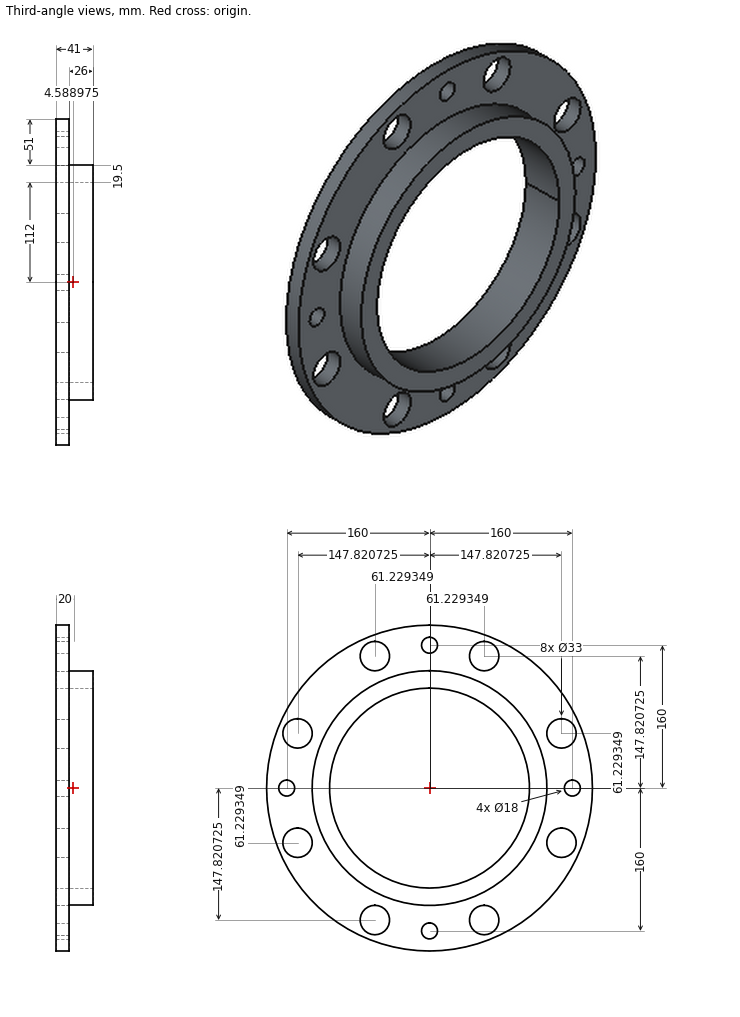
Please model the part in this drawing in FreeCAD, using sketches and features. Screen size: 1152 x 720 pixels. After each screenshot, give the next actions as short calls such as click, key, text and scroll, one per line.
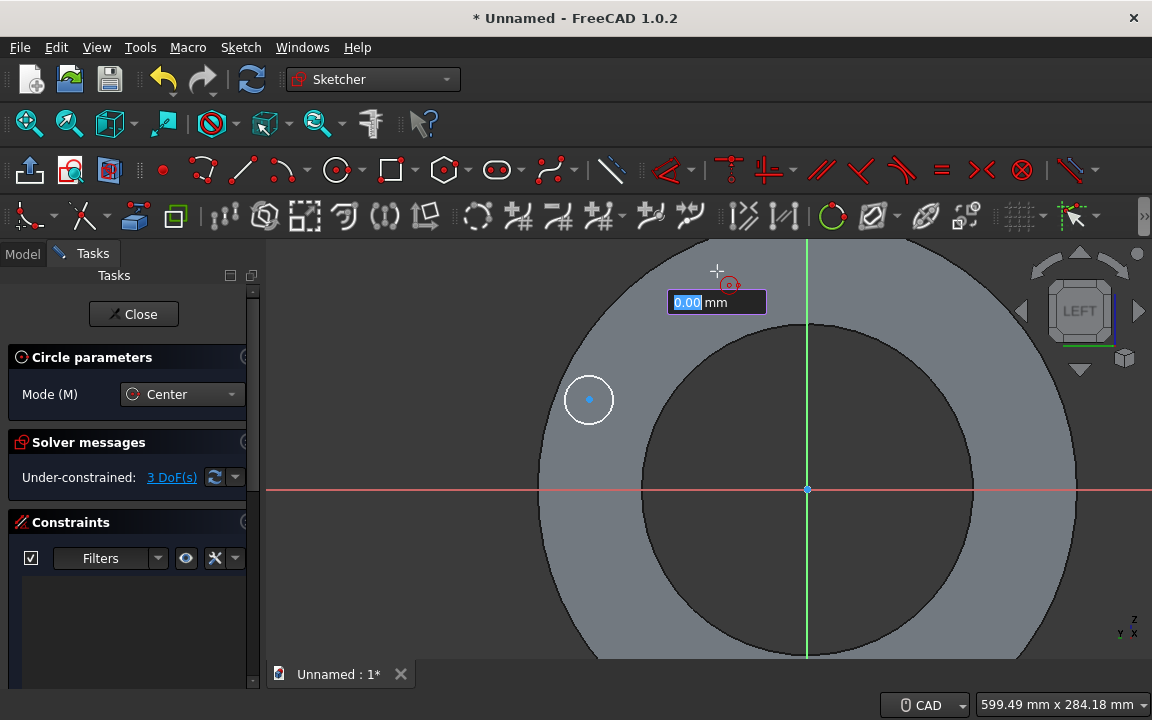
scroll(438, 399, down, 3)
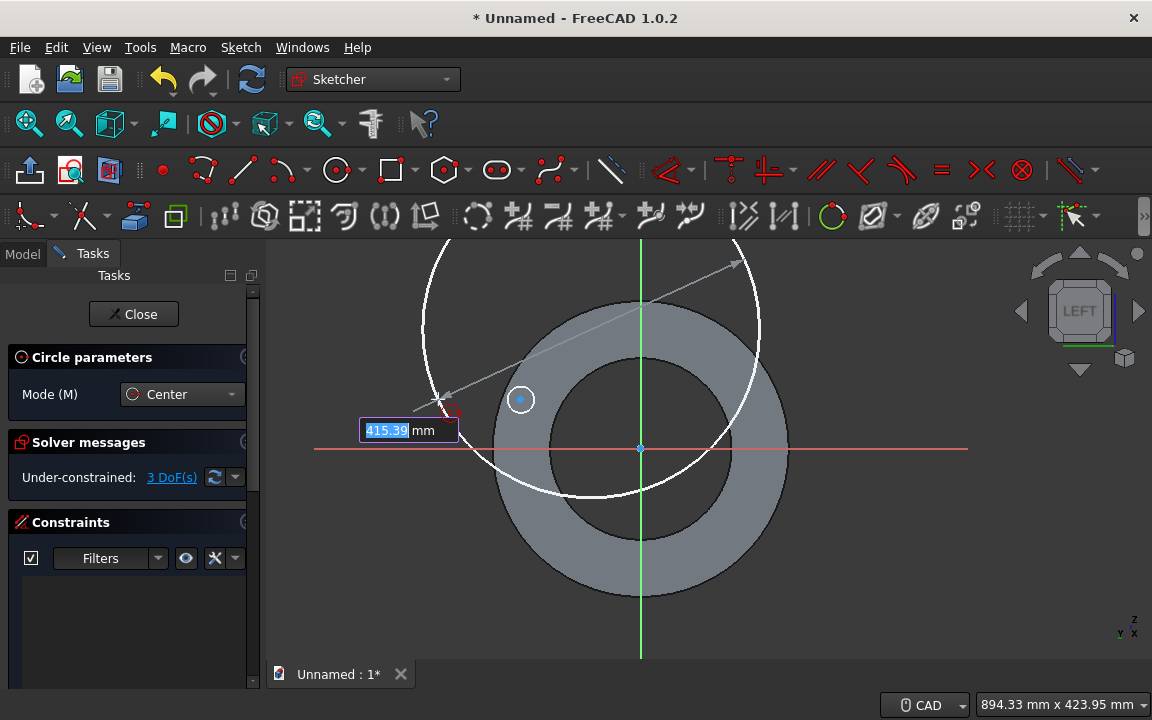
click(601, 320)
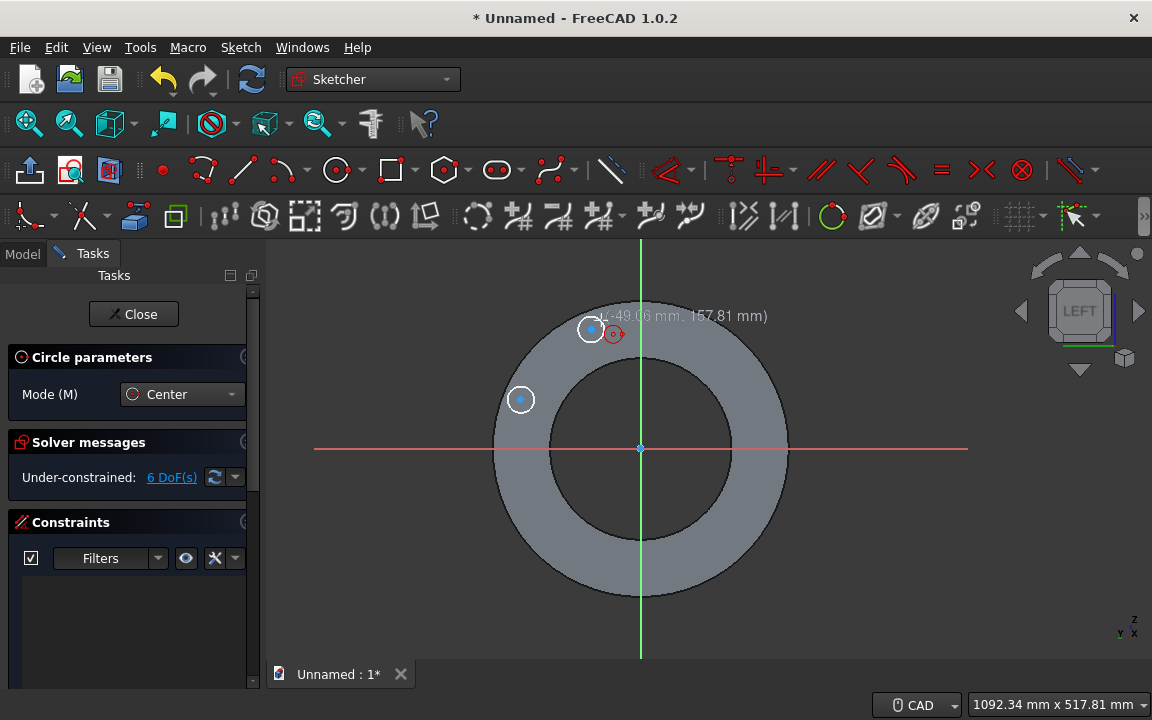
scroll(690, 329, up, 3)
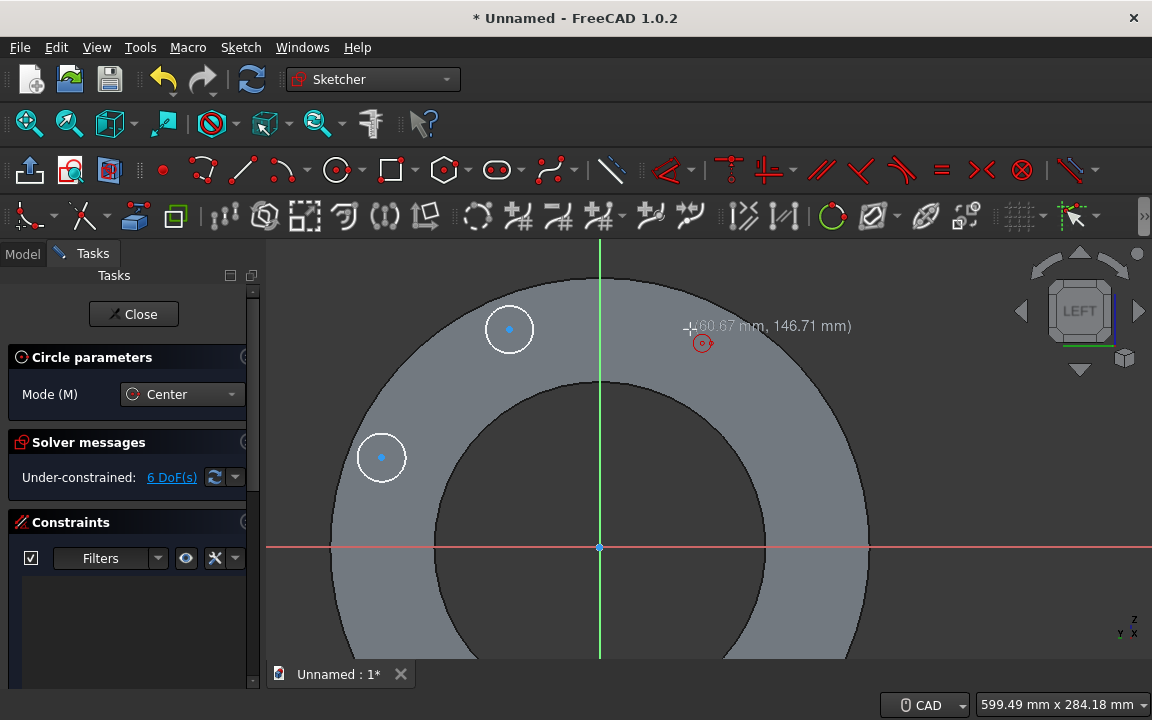
click(690, 329)
click(708, 312)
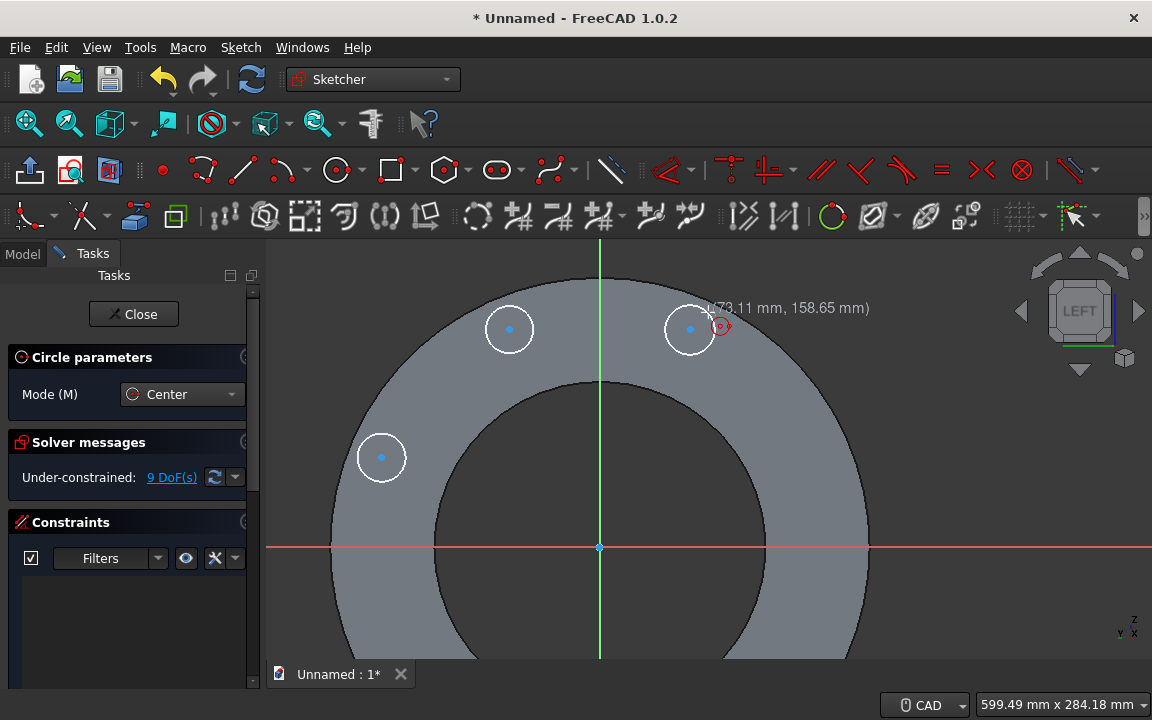
click(818, 457)
click(836, 440)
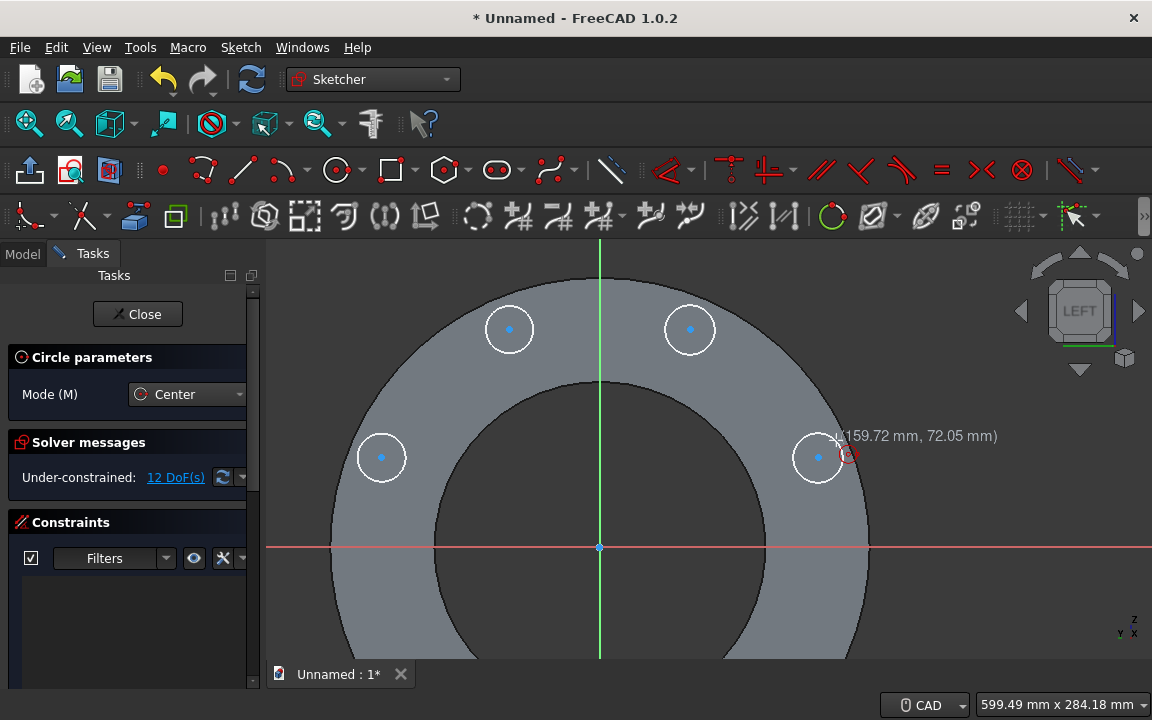
scroll(690, 329, down, 3)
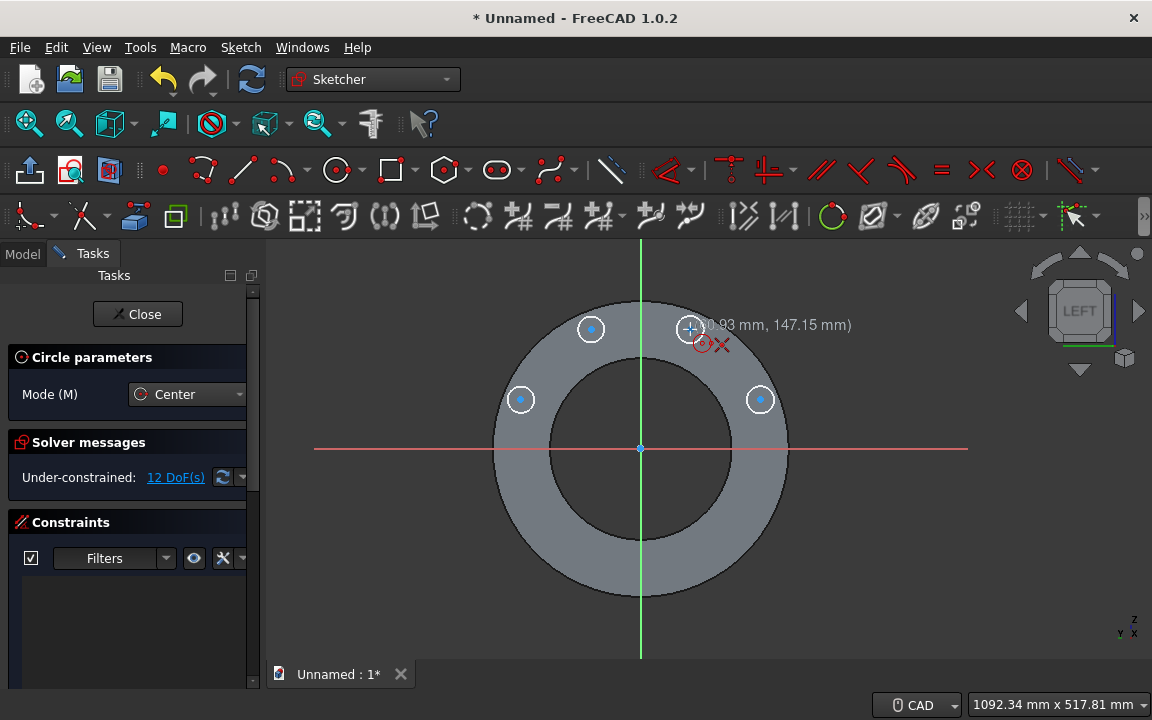
scroll(761, 499, up, 3)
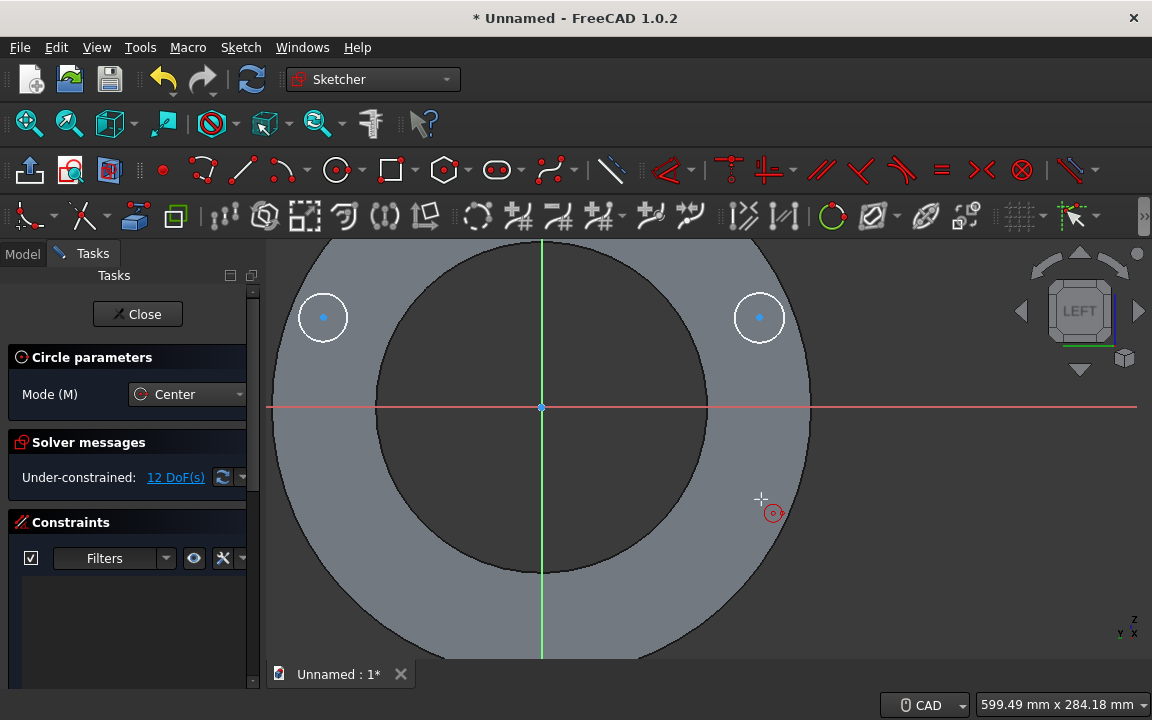
click(760, 498)
click(777, 481)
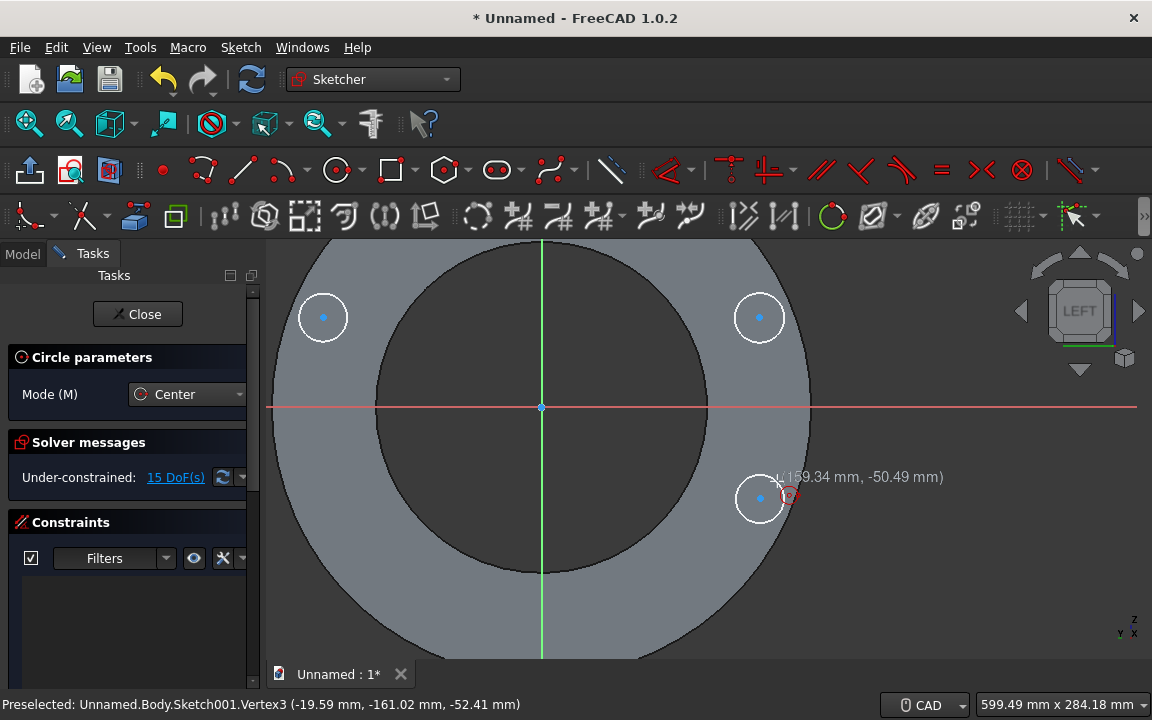
click(632, 626)
click(649, 609)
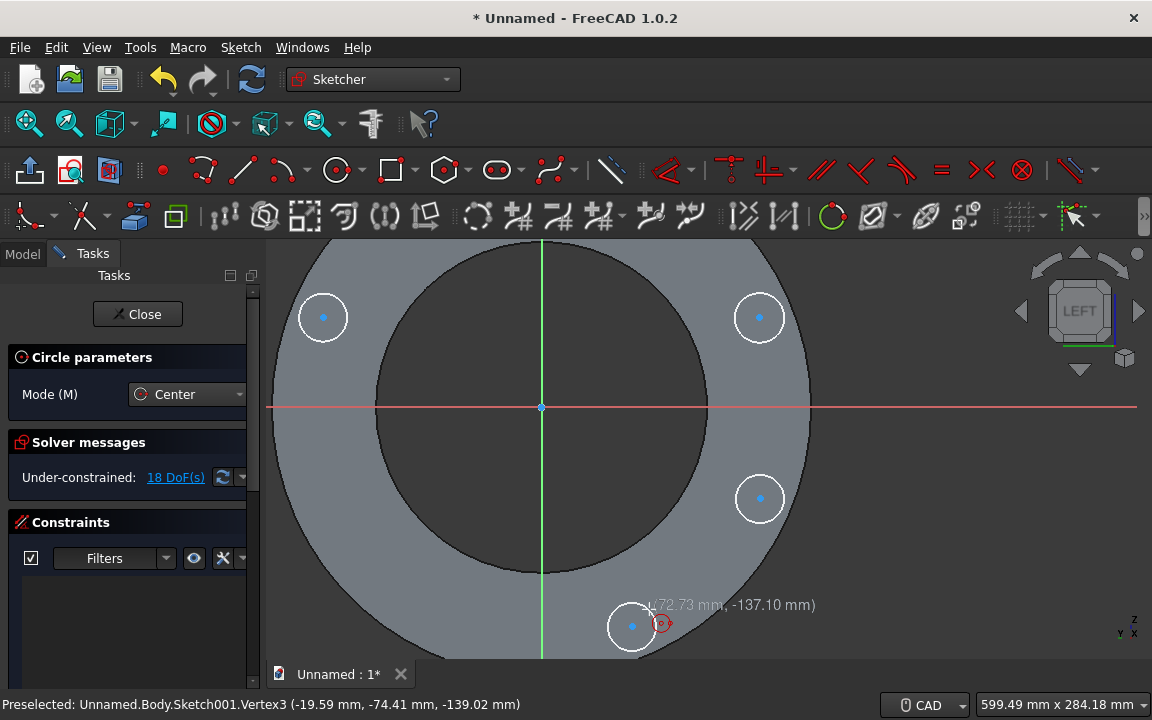
click(451, 626)
click(468, 609)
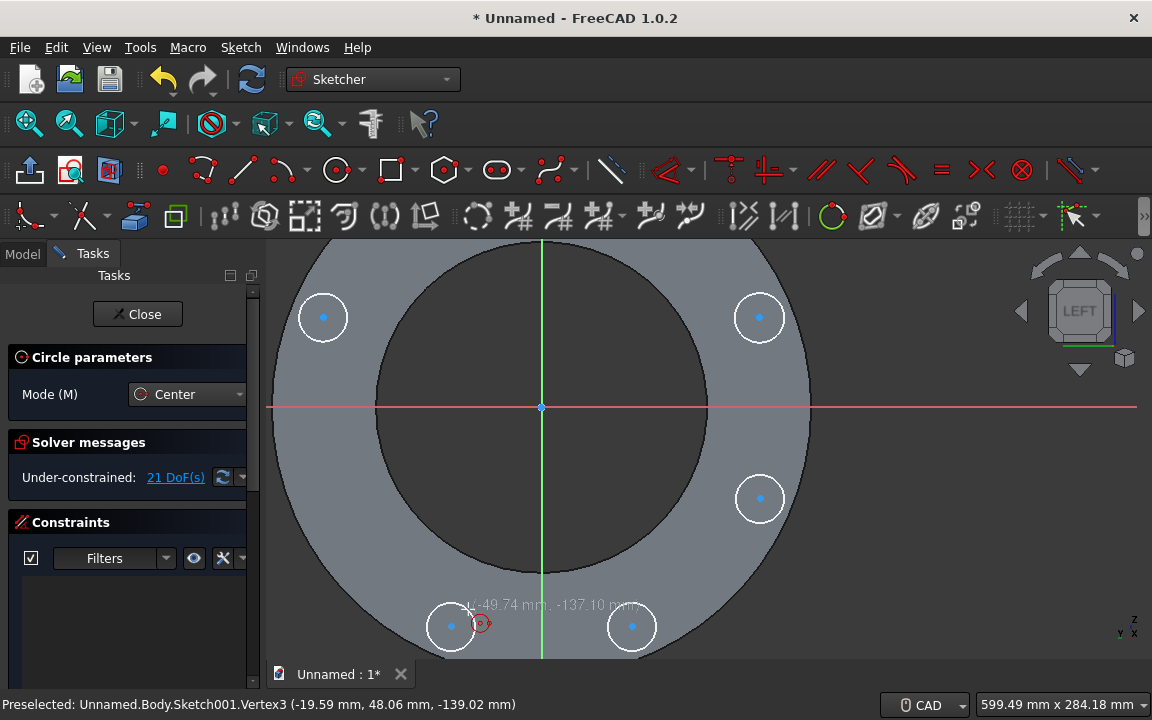
click(323, 498)
click(340, 481)
key(Escape)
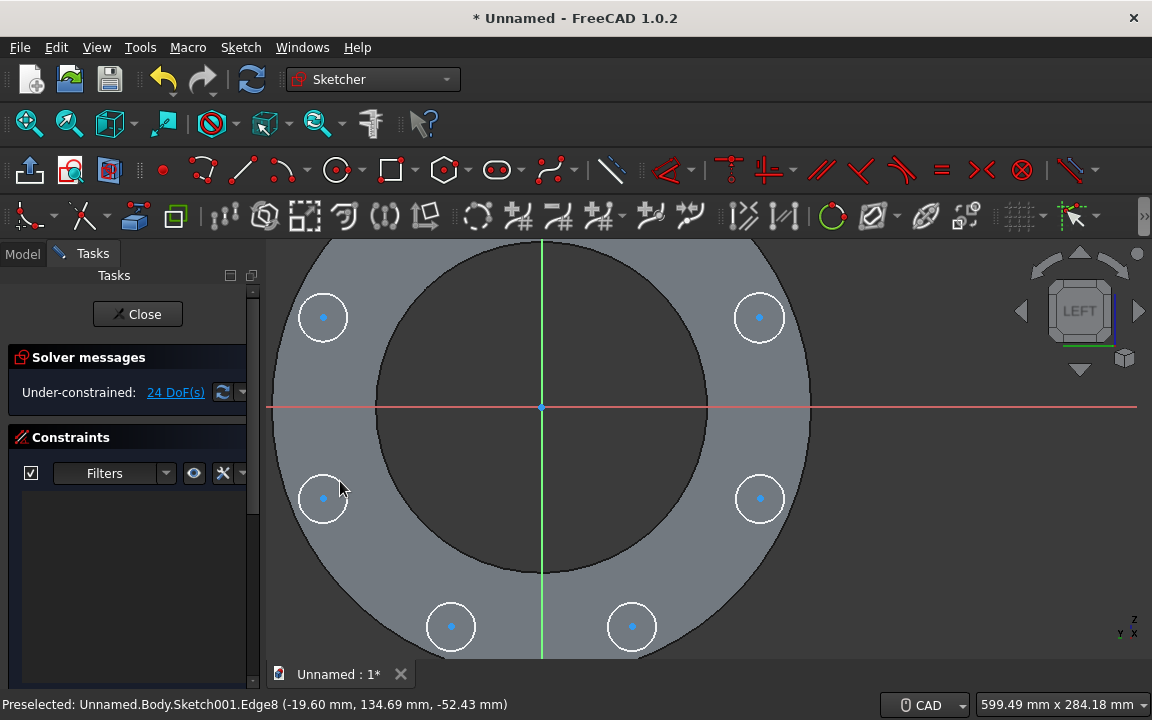
click(340, 301)